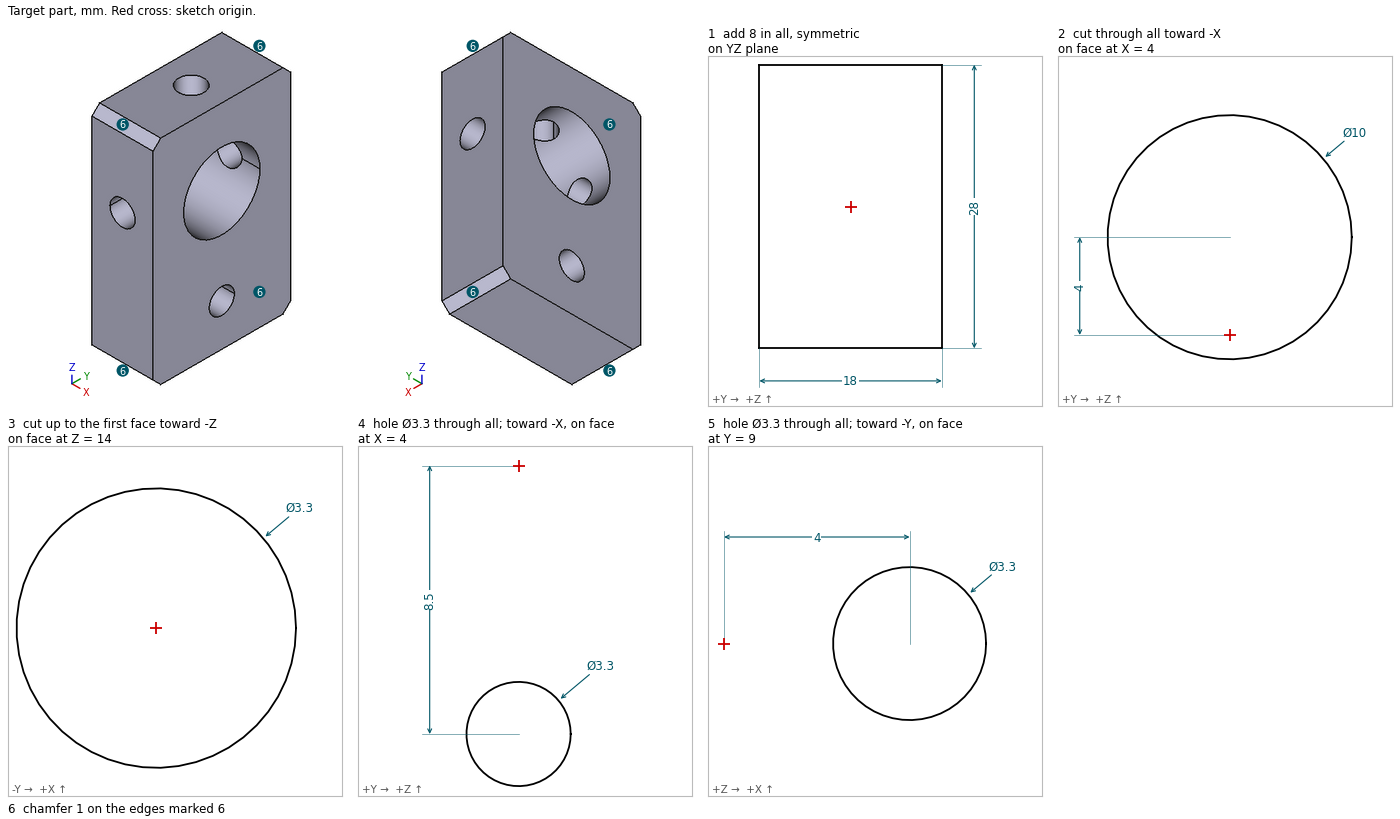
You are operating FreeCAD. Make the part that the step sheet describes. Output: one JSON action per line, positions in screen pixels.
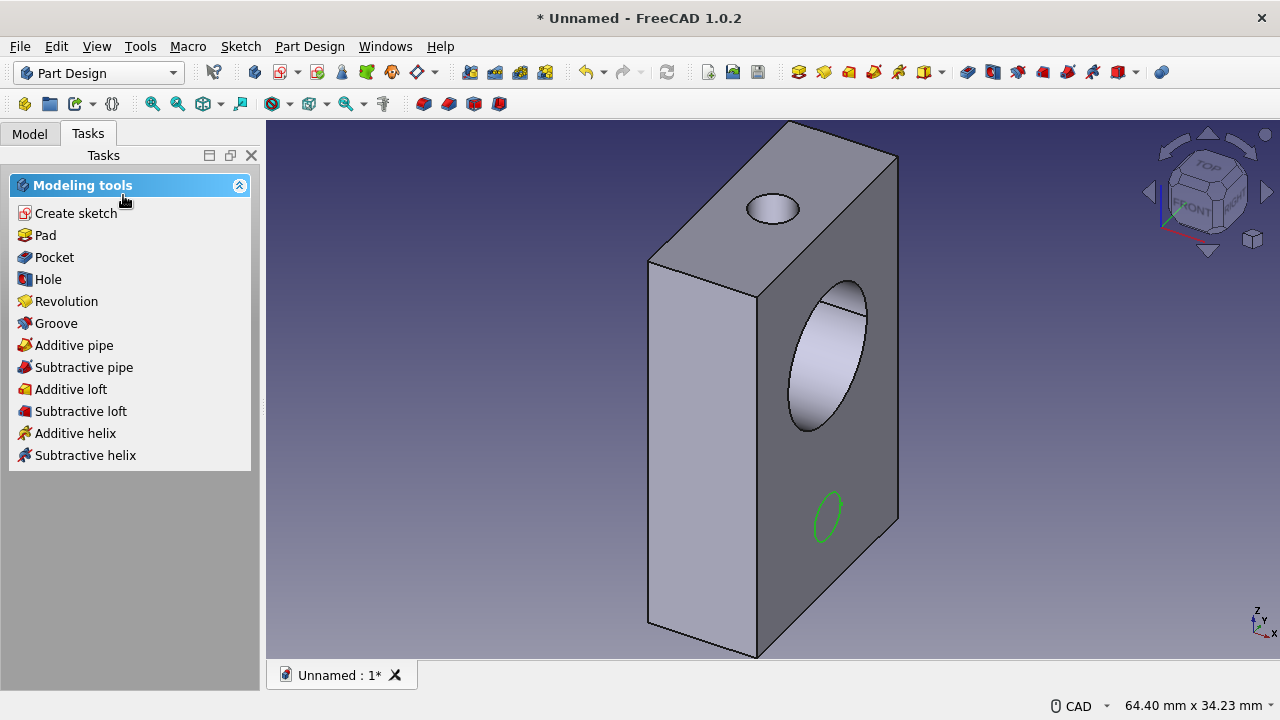
{"action": "left_click", "coordinate": [993, 72]}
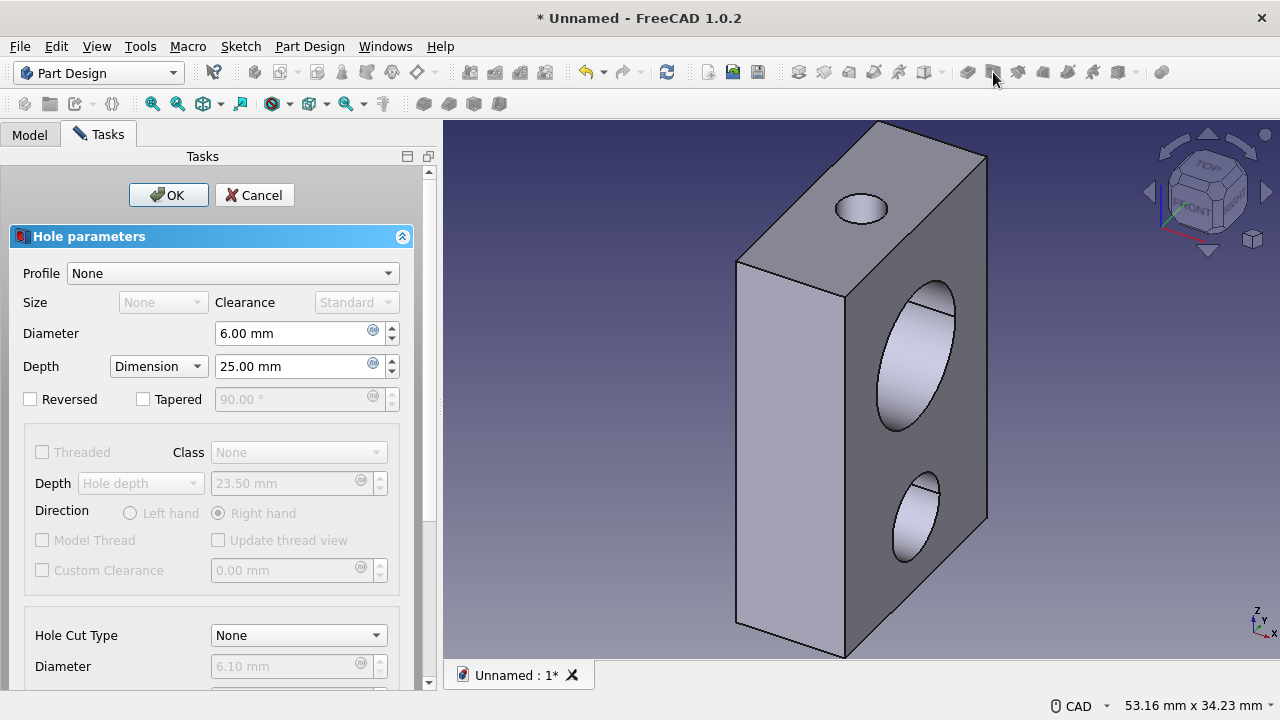
{"action": "triple_click", "coordinate": [300, 334]}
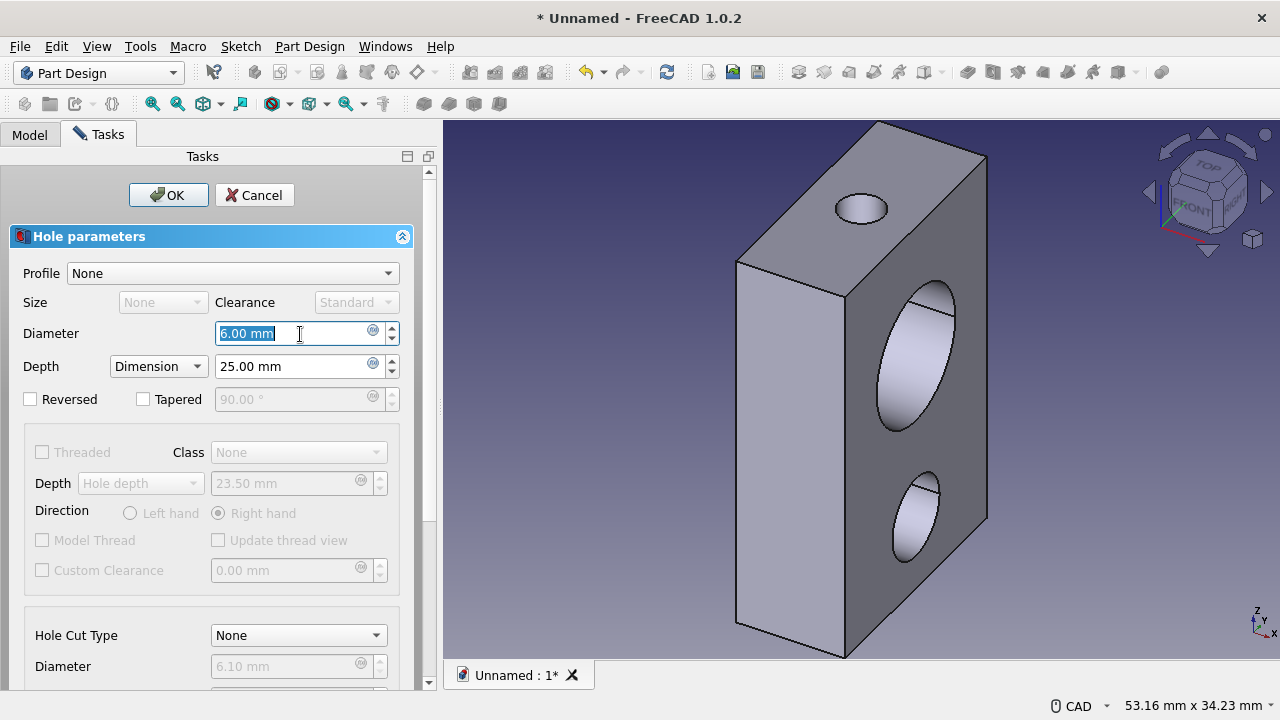
{"action": "type", "text": "3.3"}
{"action": "key", "text": "Tab"}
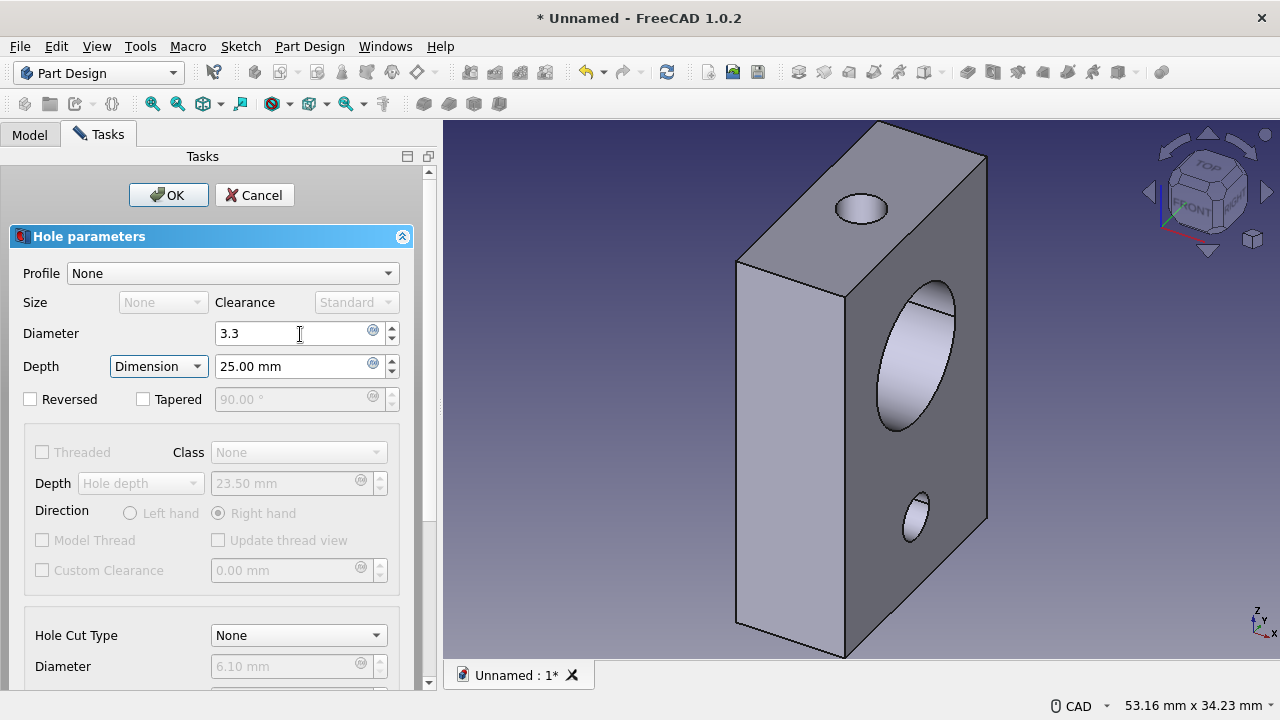
{"action": "left_click", "coordinate": [160, 366]}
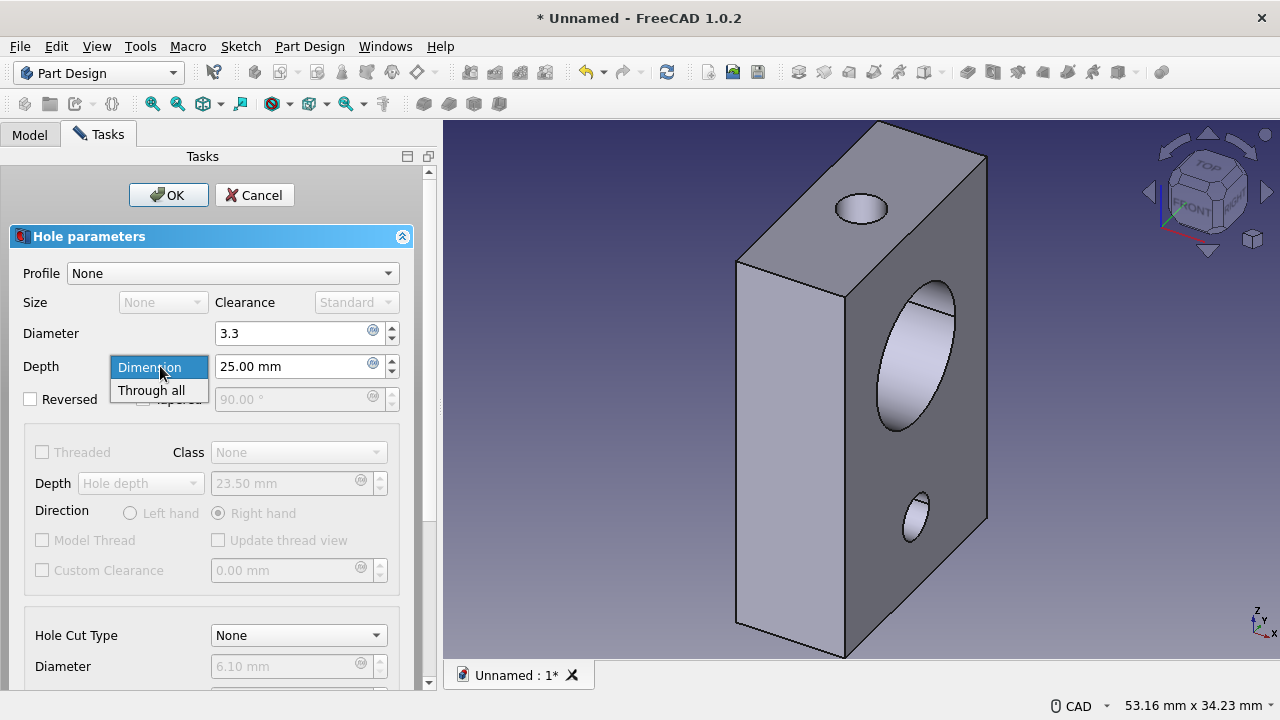
{"action": "left_click", "coordinate": [158, 390]}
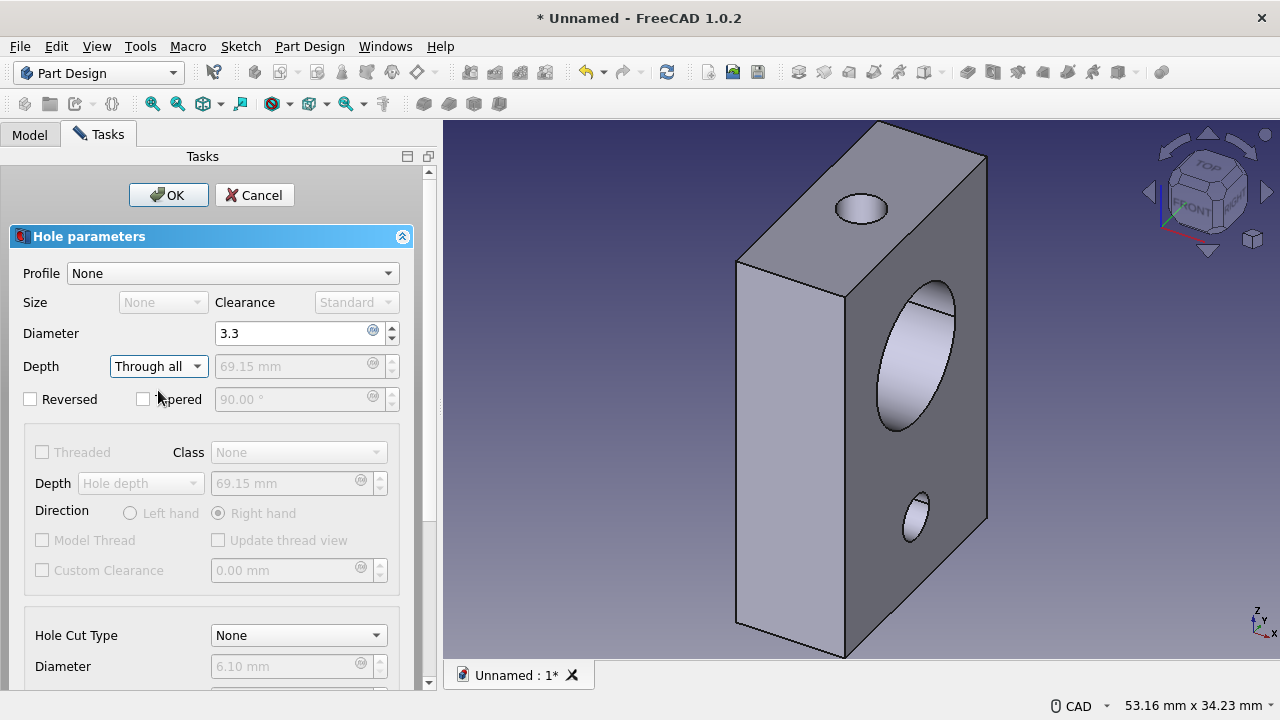
{"action": "left_click", "coordinate": [169, 195]}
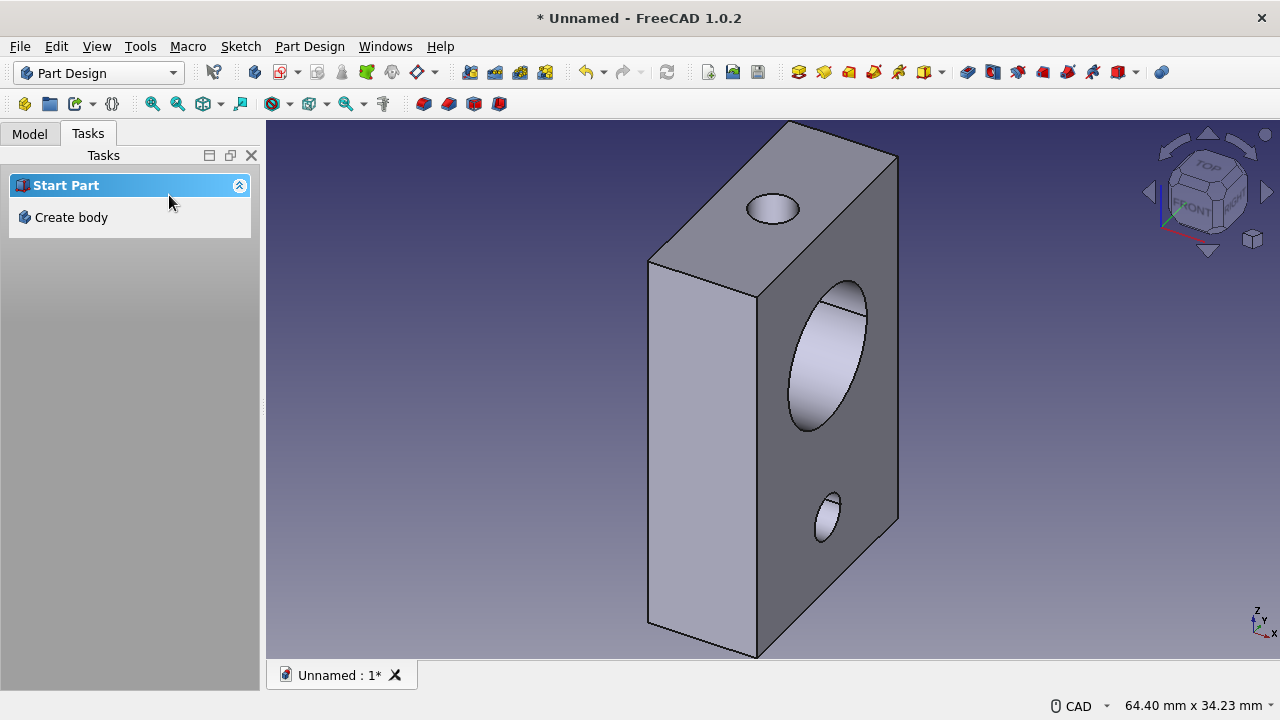
{"action": "left_click", "coordinate": [153, 104]}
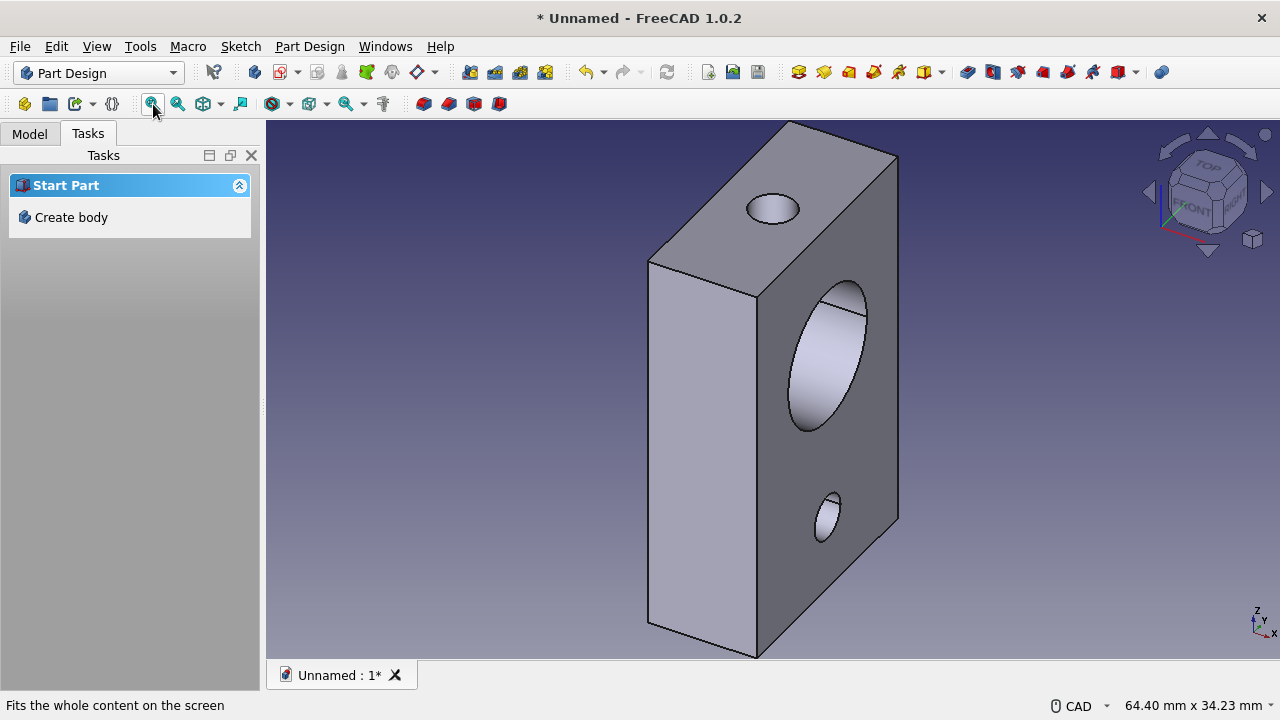
{"action": "key", "text": "4"}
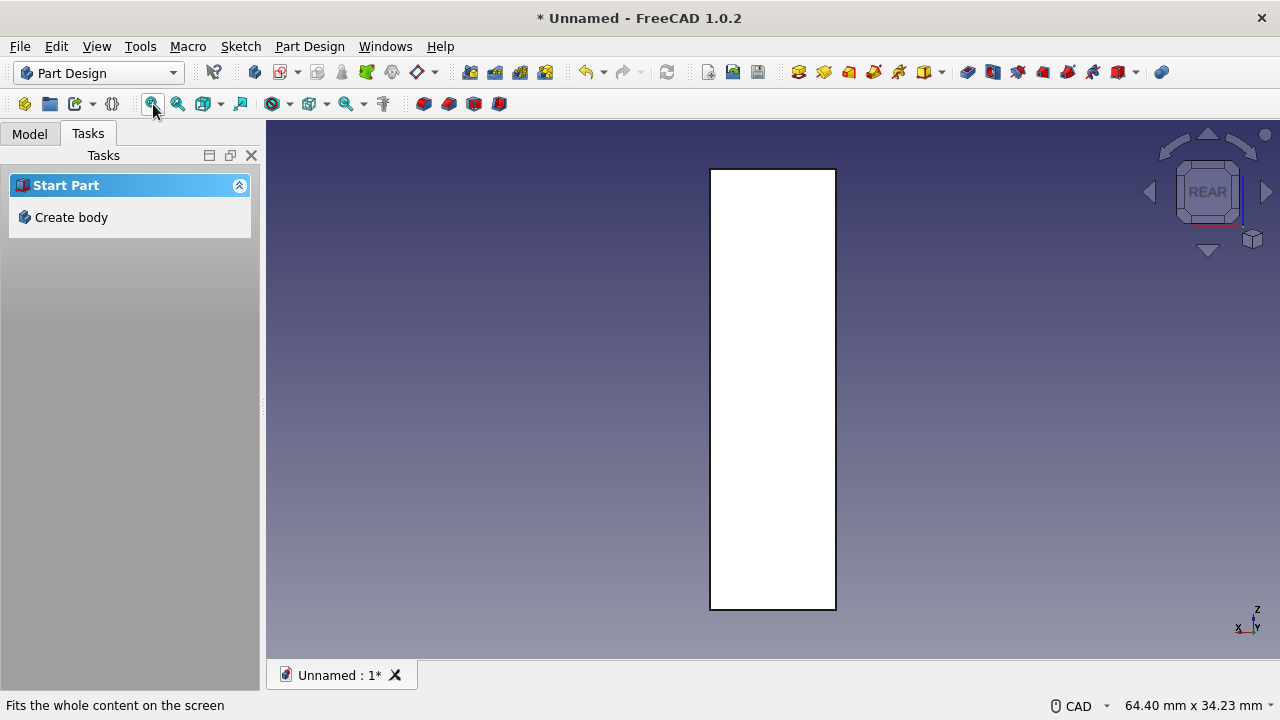
{"action": "left_click", "coordinate": [773, 514]}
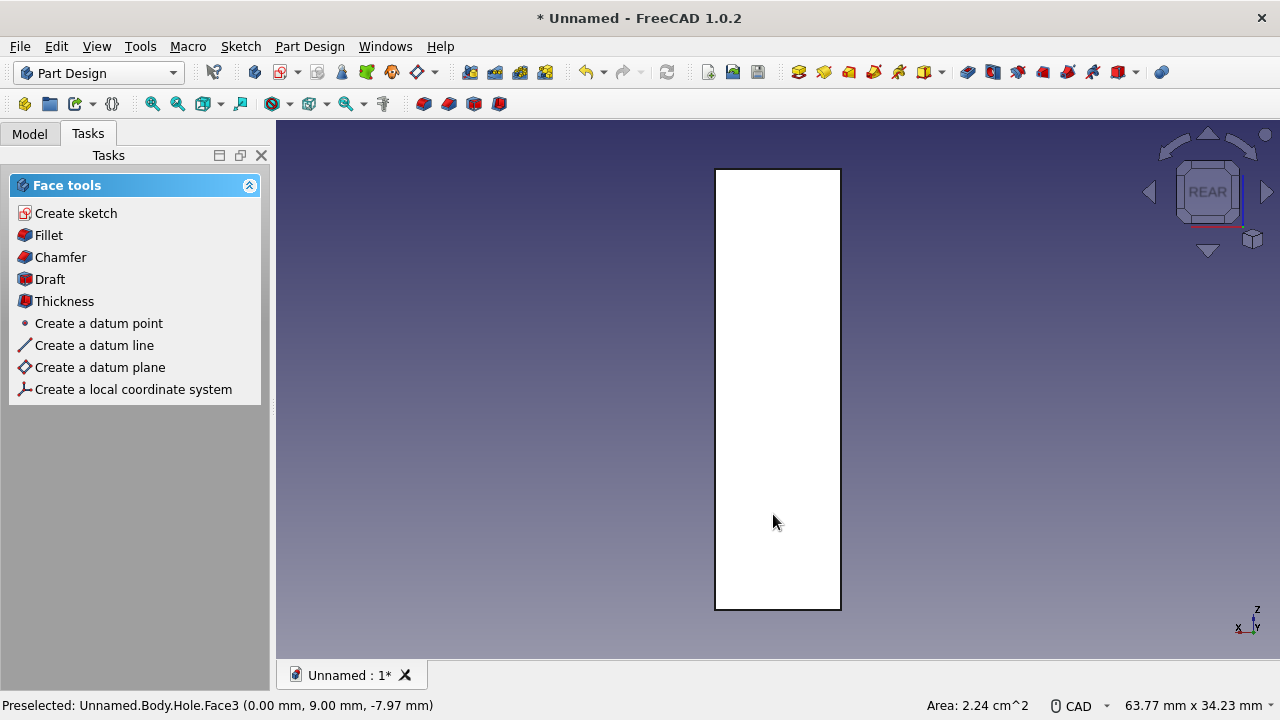
{"action": "left_click", "coordinate": [280, 72]}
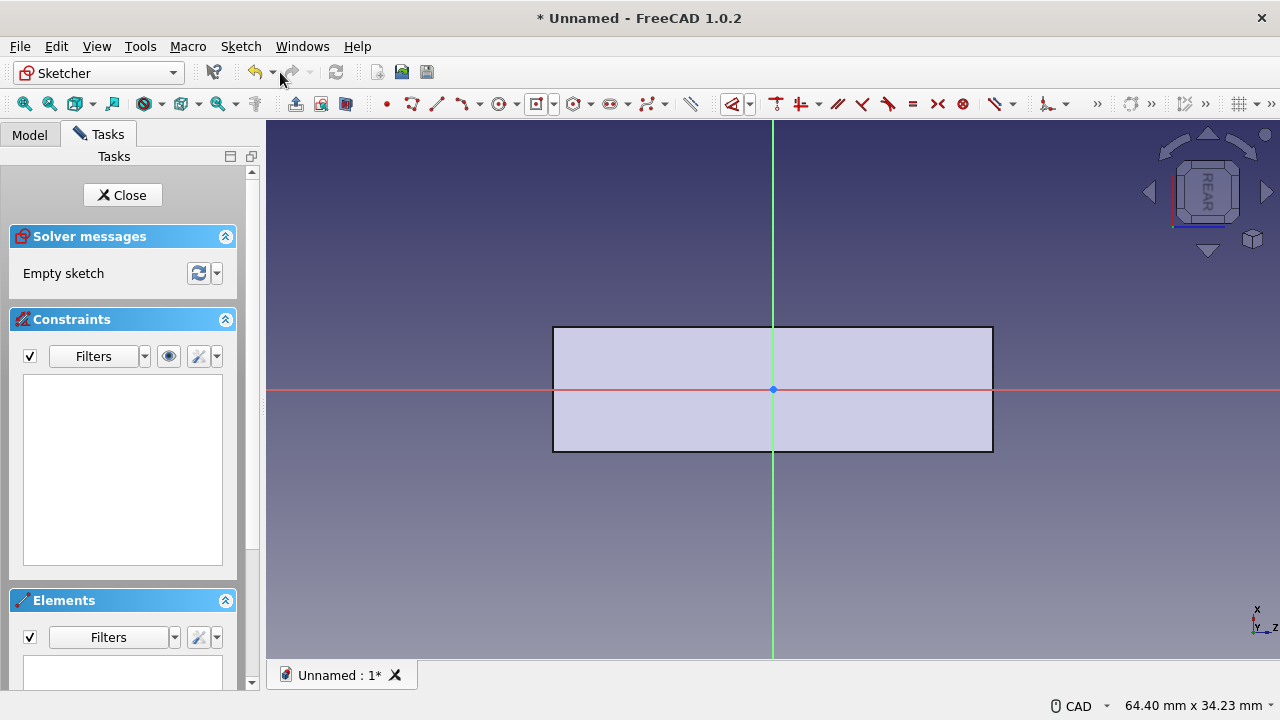
{"action": "scroll", "coordinate": [840, 390], "scroll_direction": "up", "scroll_amount": 9}